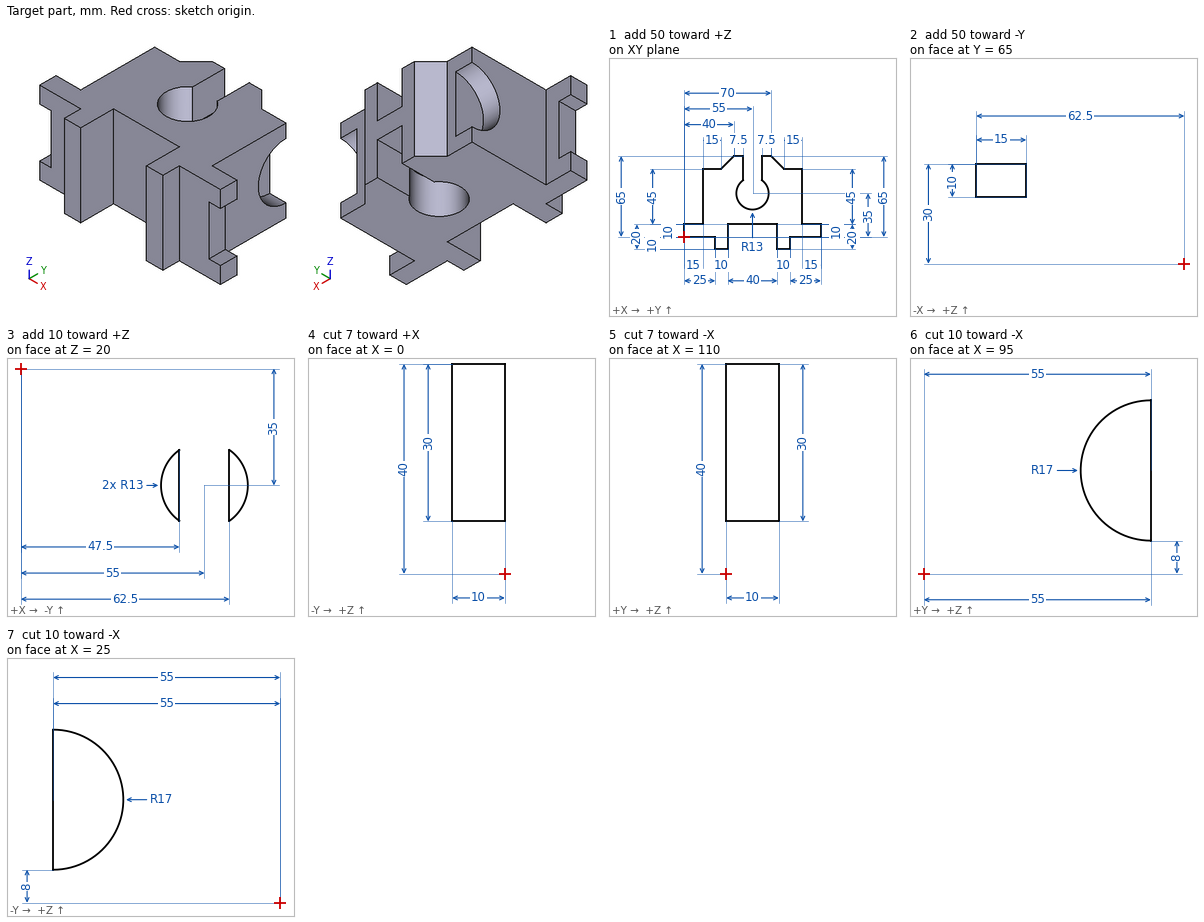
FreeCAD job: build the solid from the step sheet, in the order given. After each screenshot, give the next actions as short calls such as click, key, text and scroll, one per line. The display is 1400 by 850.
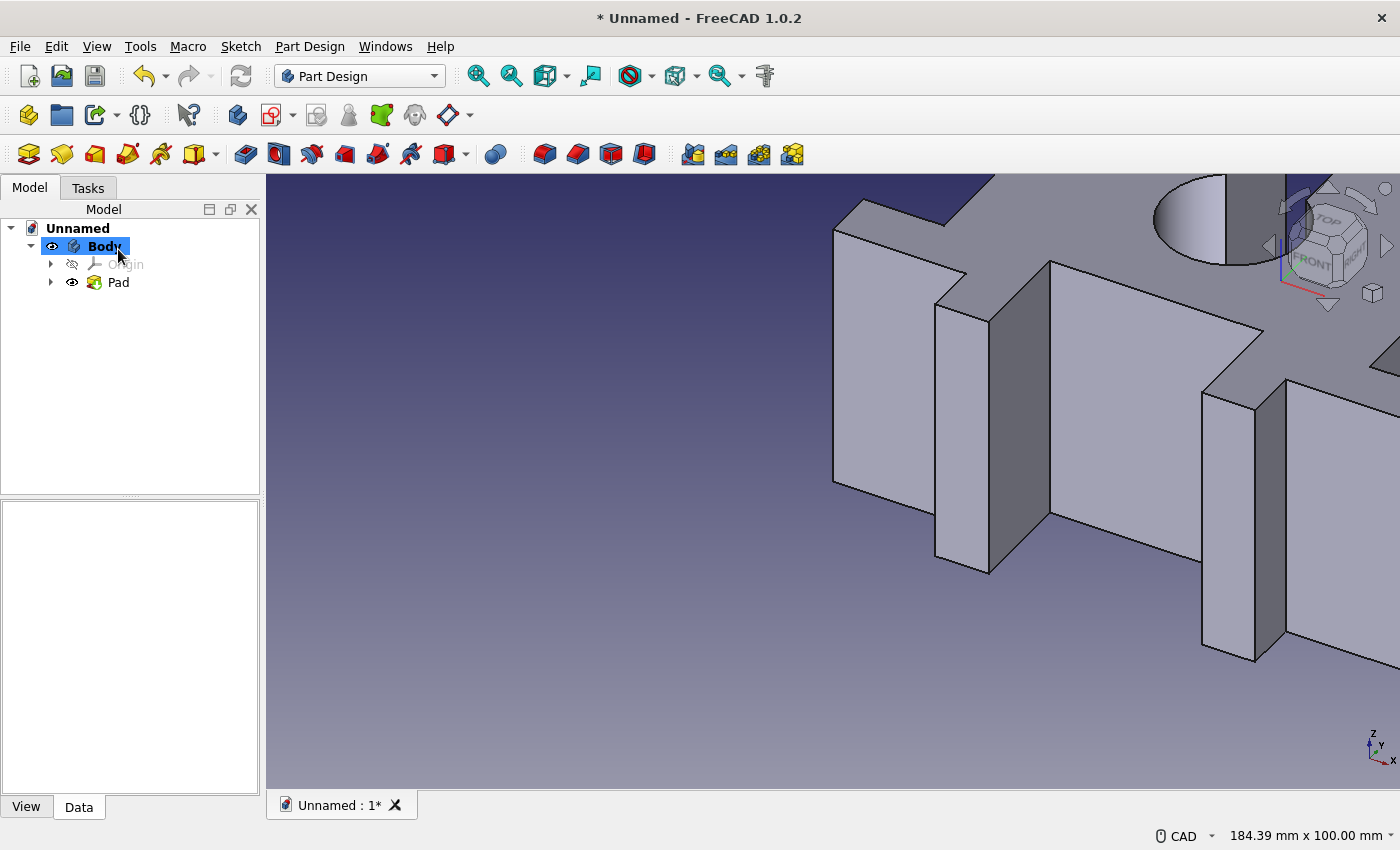
click(479, 76)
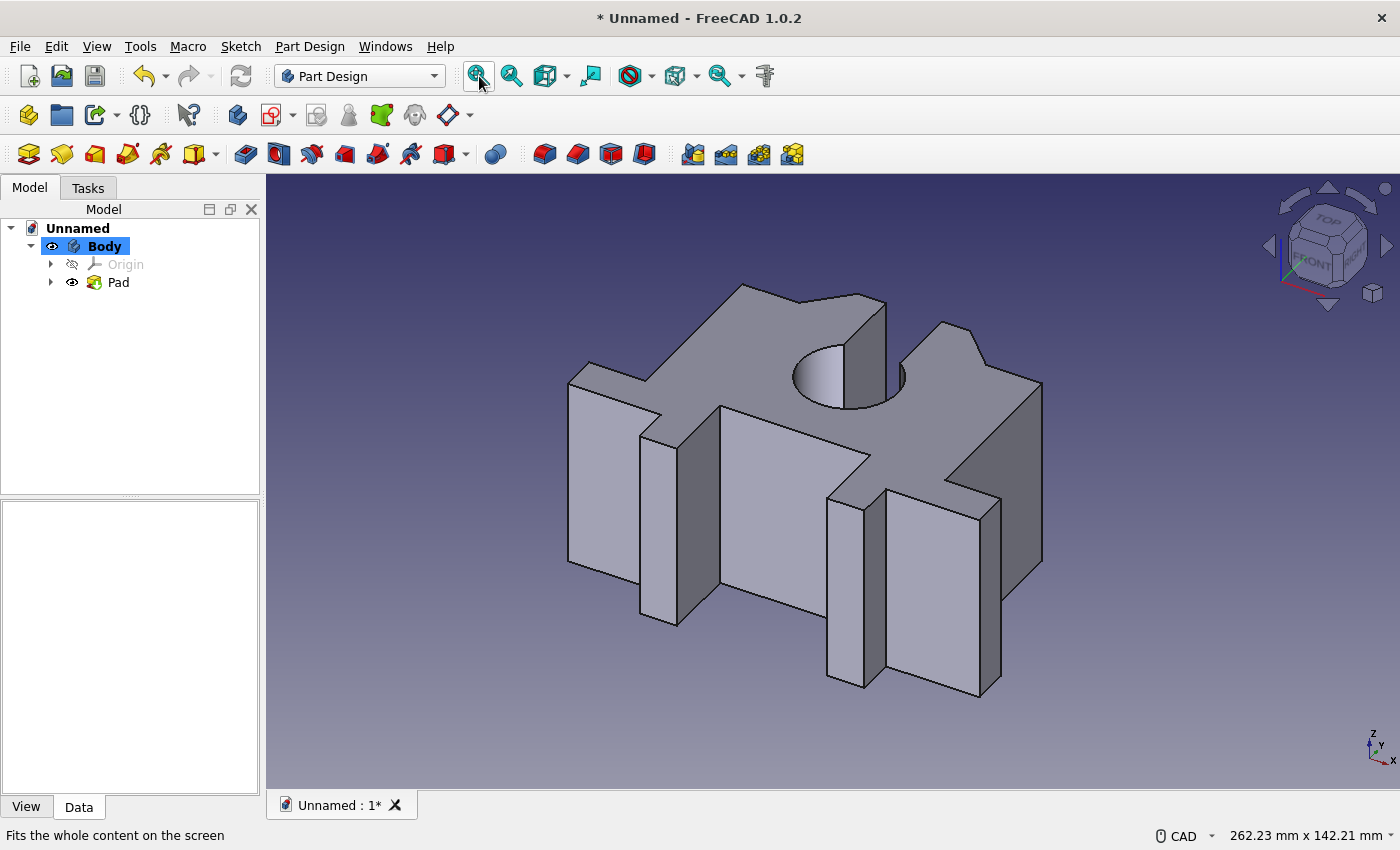
key(4)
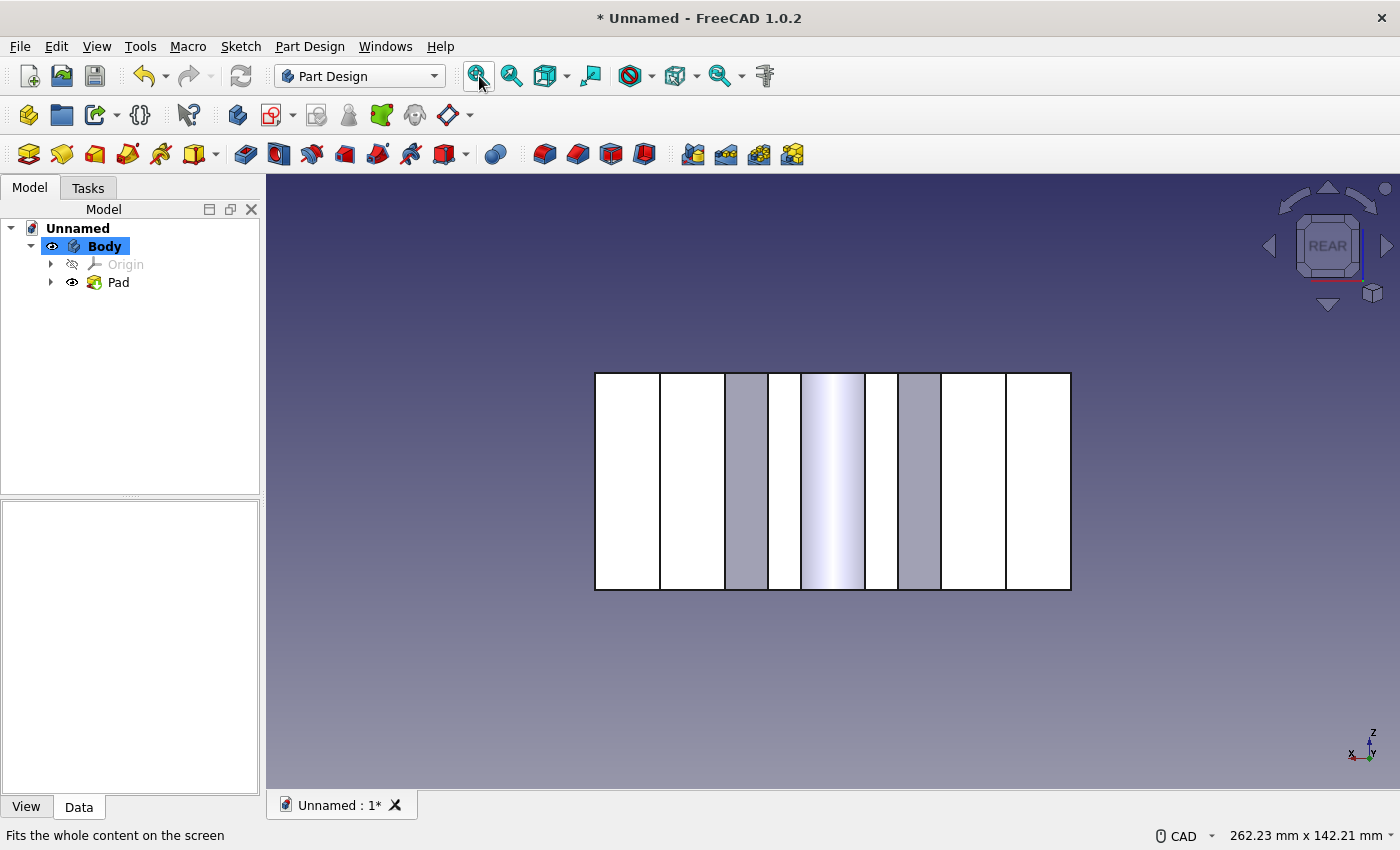
click(479, 76)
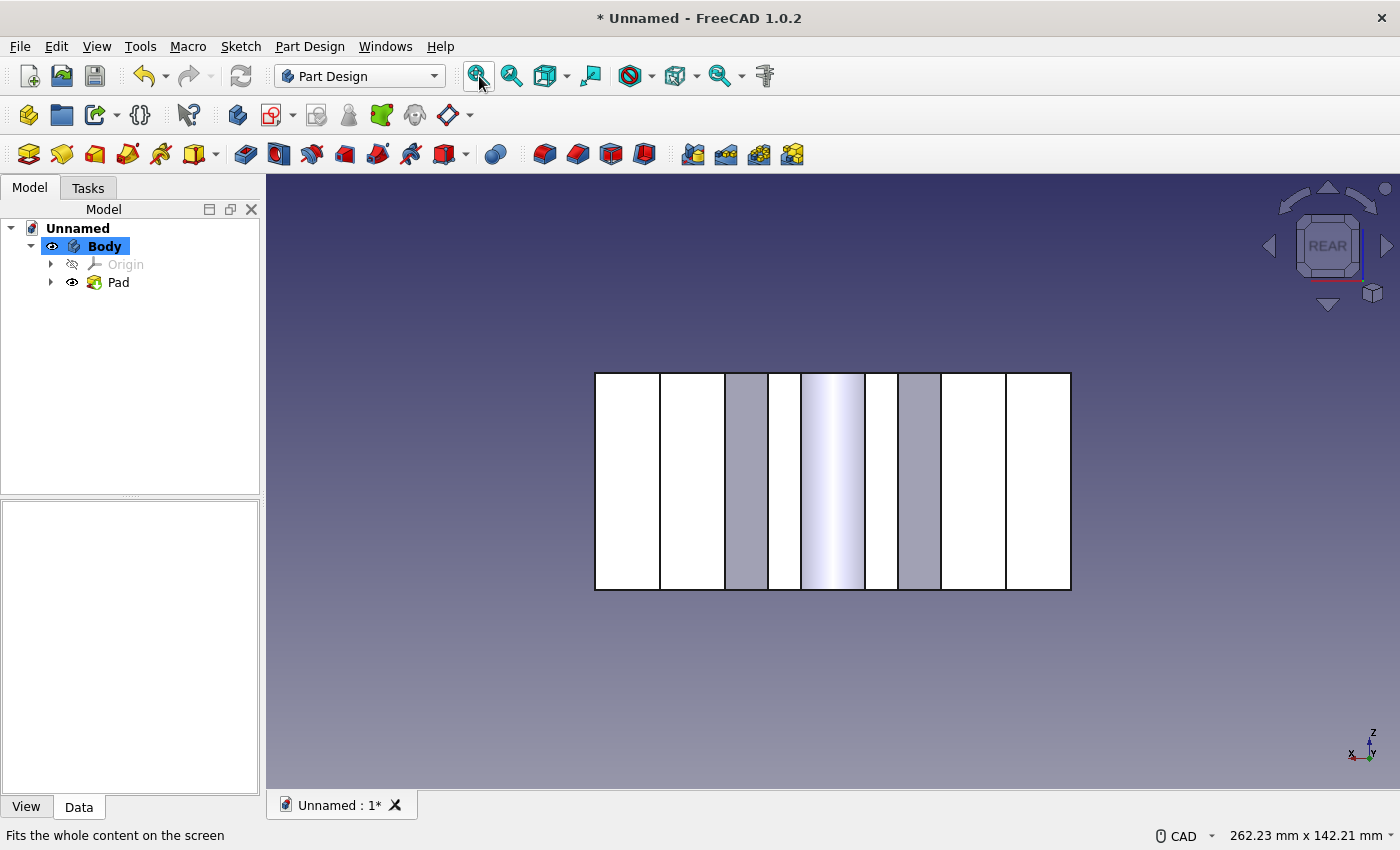
click(784, 419)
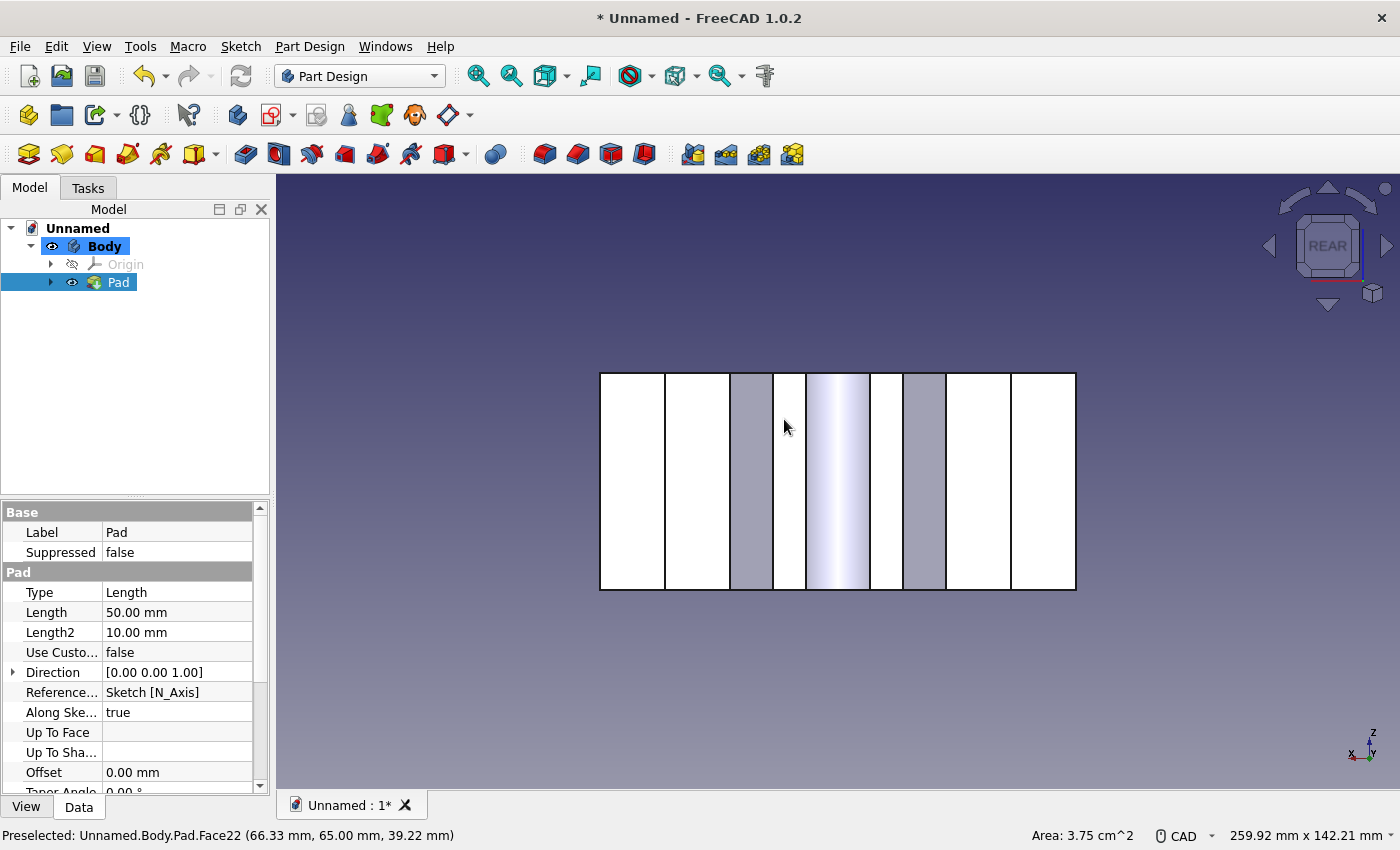
click(270, 116)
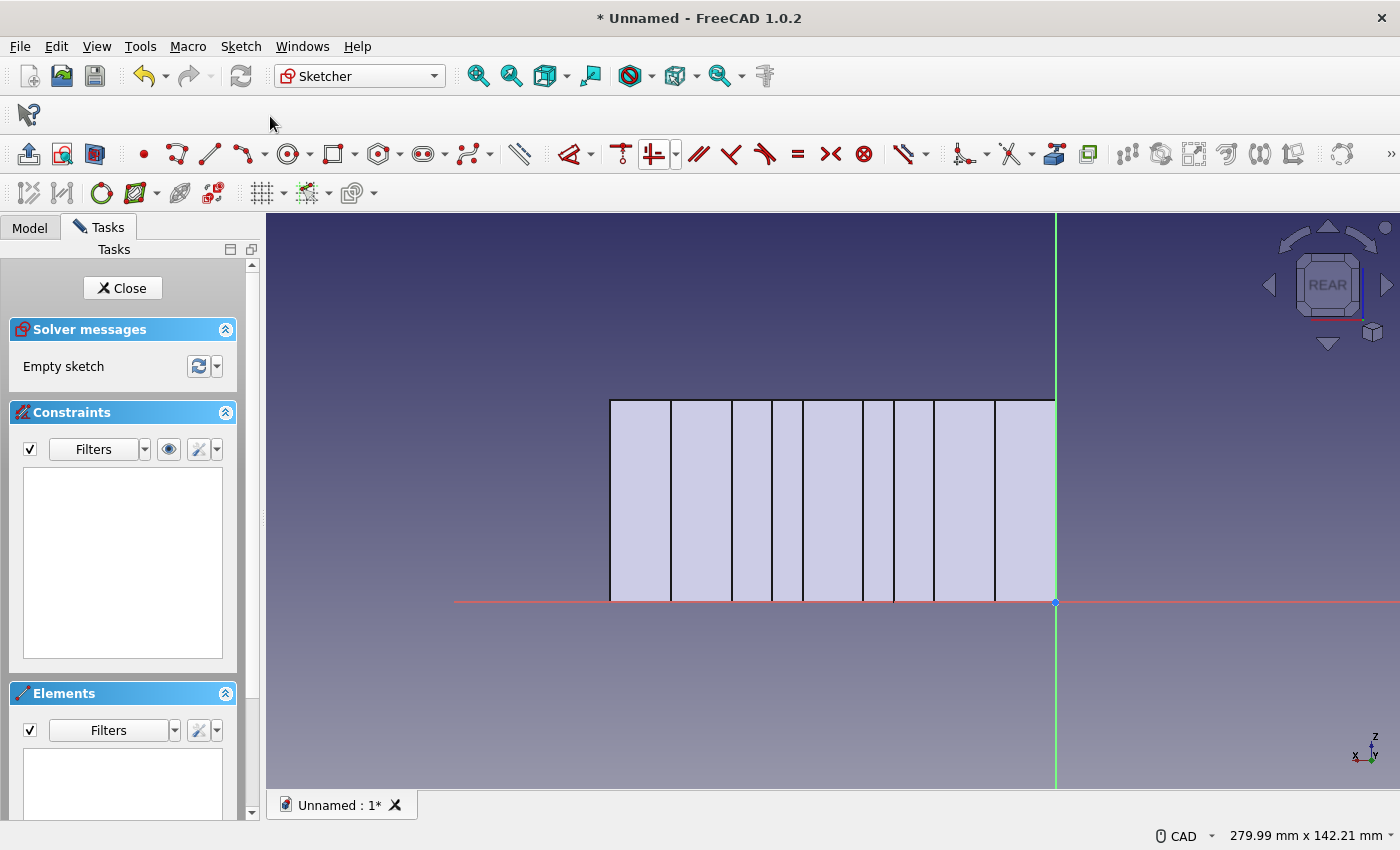
scroll(842, 501, up, 11)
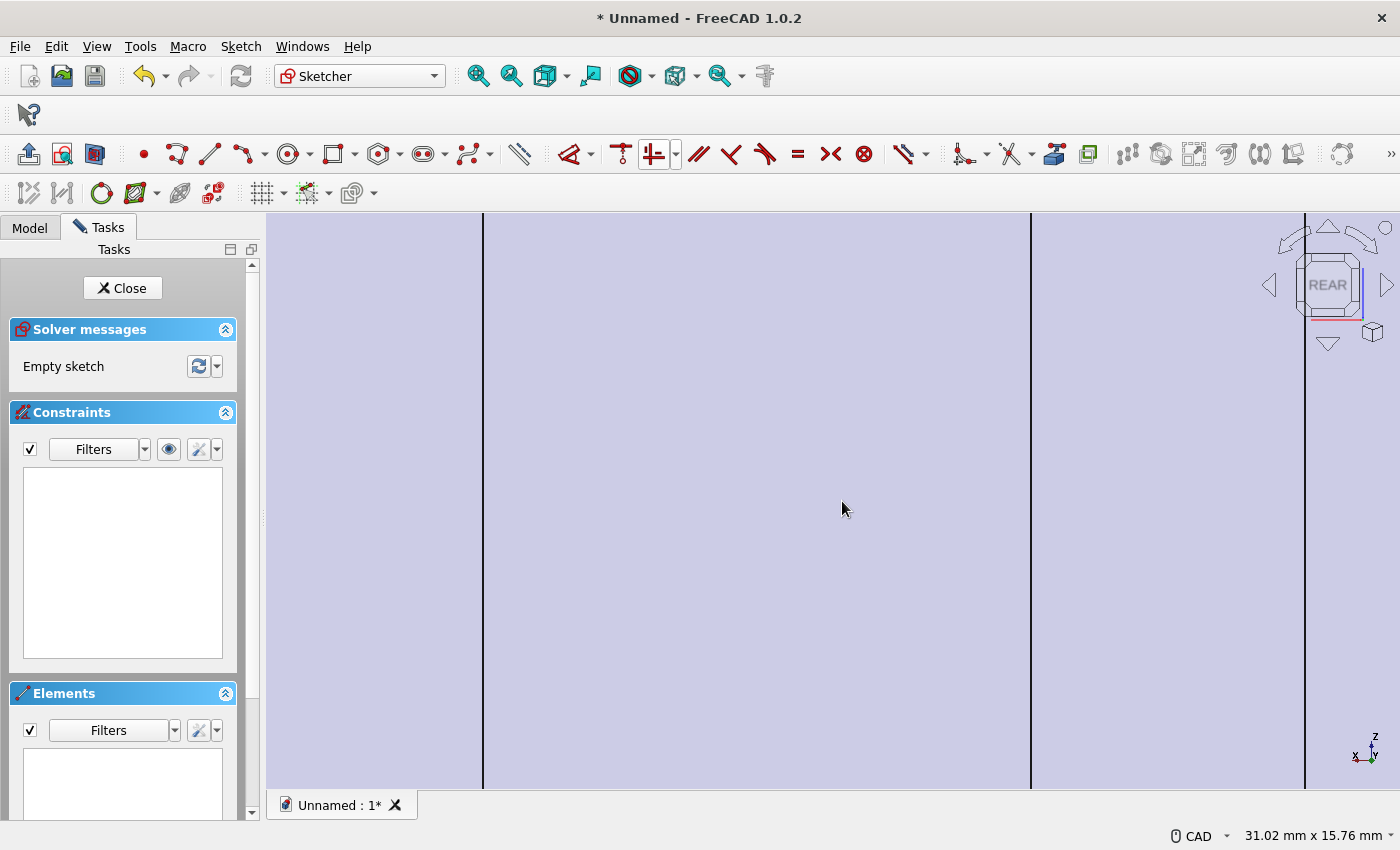
click(332, 154)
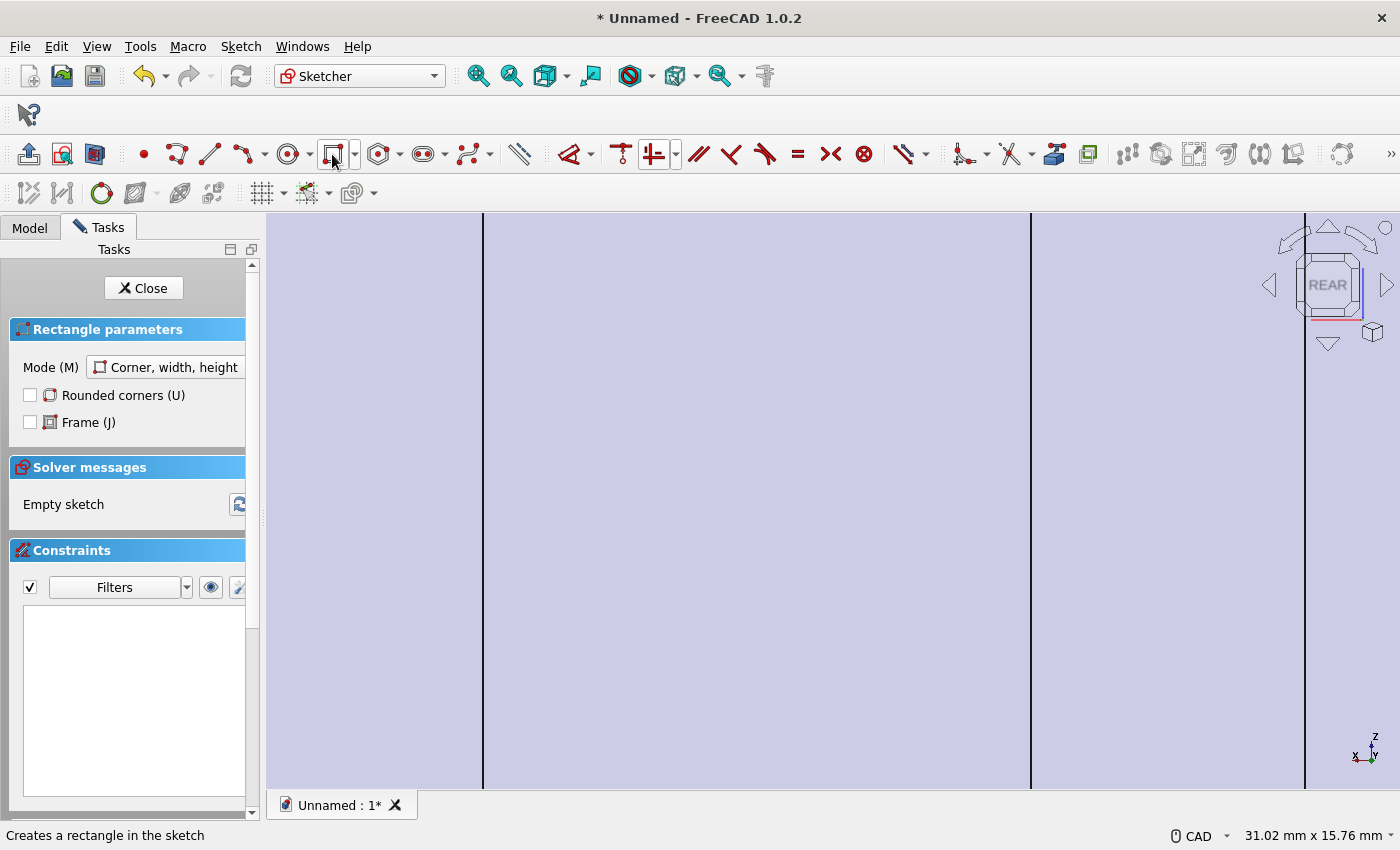
click(483, 314)
move(1031, 680)